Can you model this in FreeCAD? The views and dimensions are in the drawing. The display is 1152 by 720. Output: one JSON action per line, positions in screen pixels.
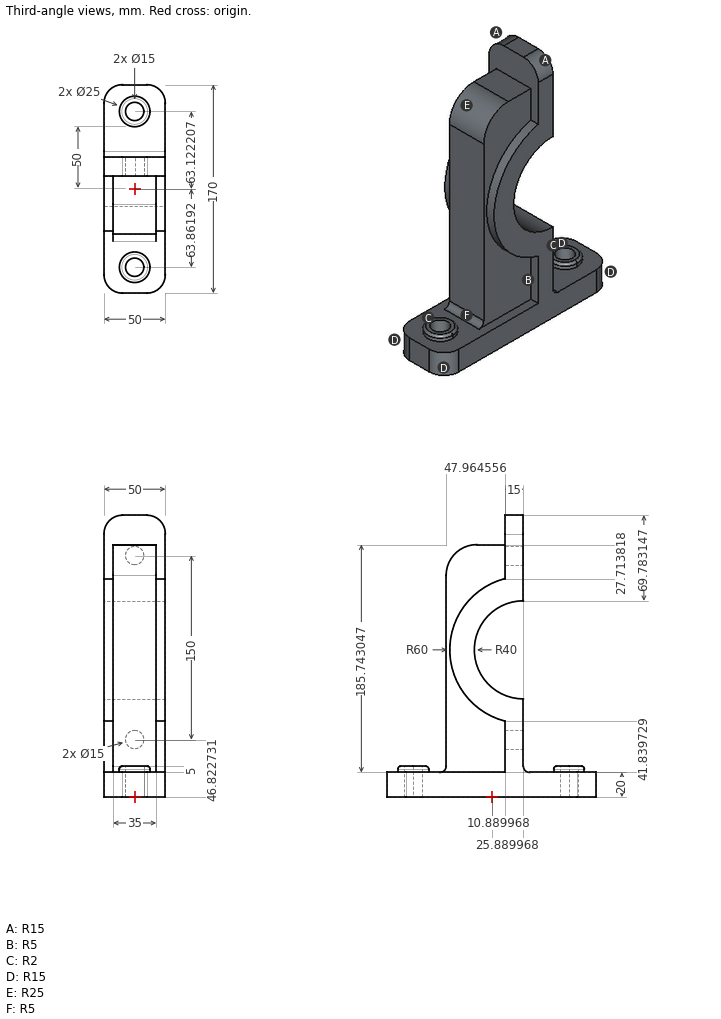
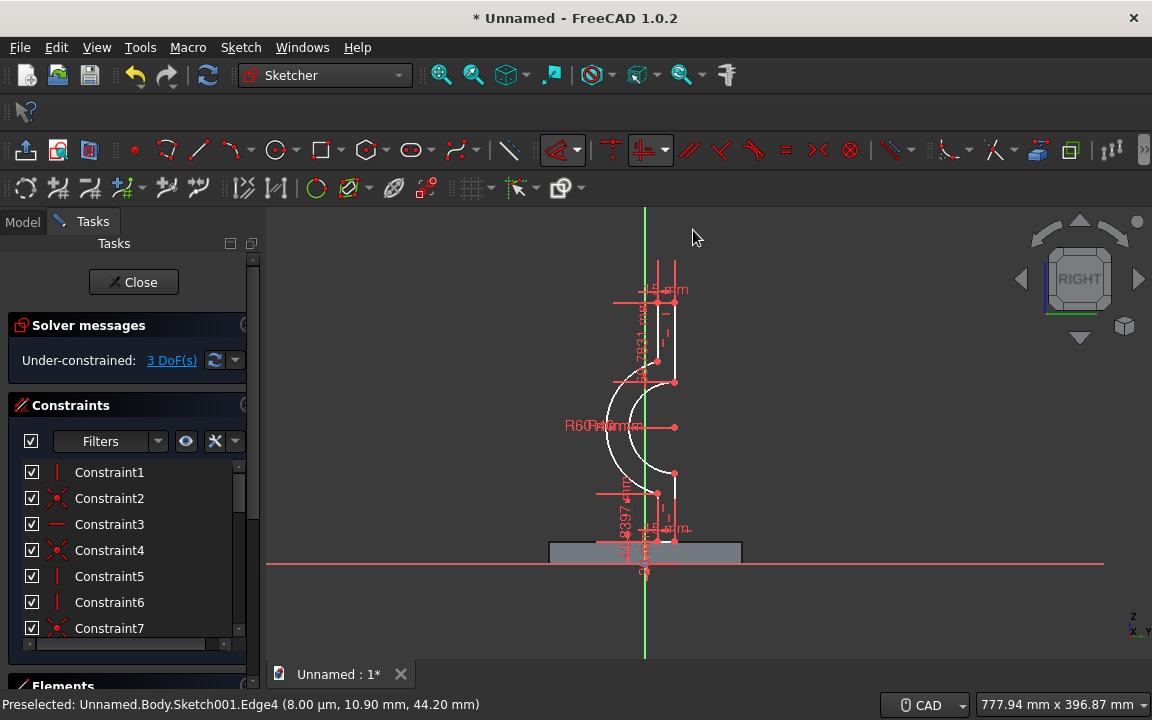
{"action": "scroll", "coordinate": [675, 382], "scroll_direction": "up", "scroll_amount": 2}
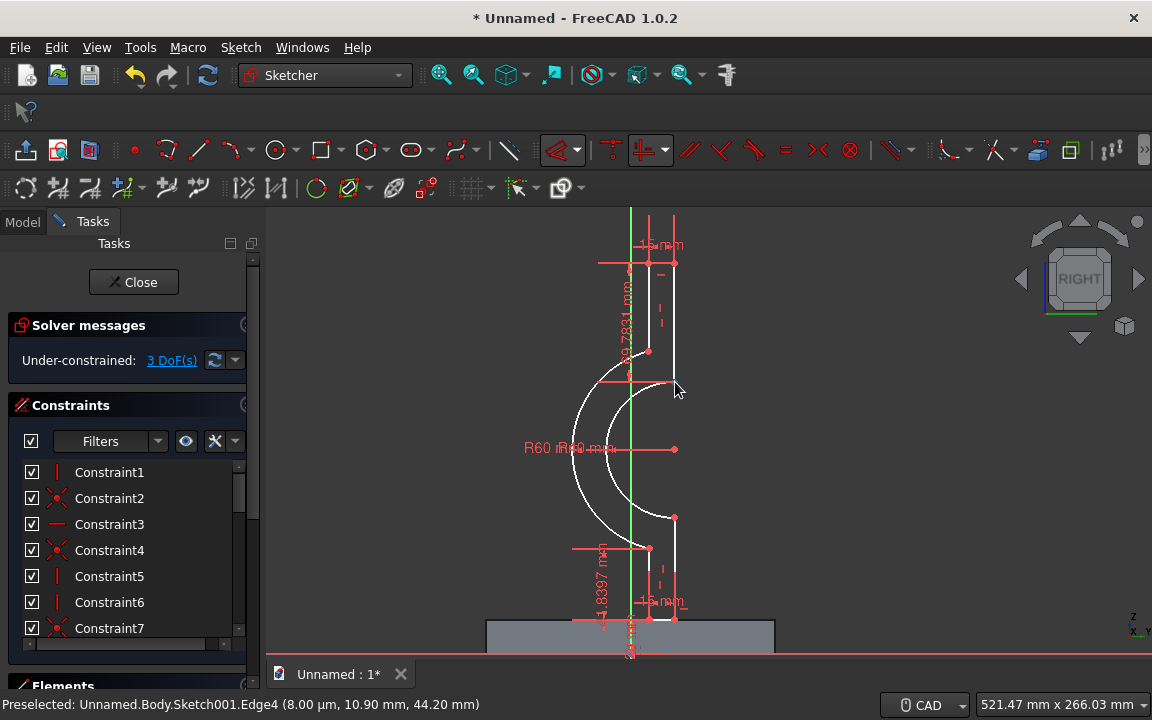
{"action": "left_click", "coordinate": [674, 382]}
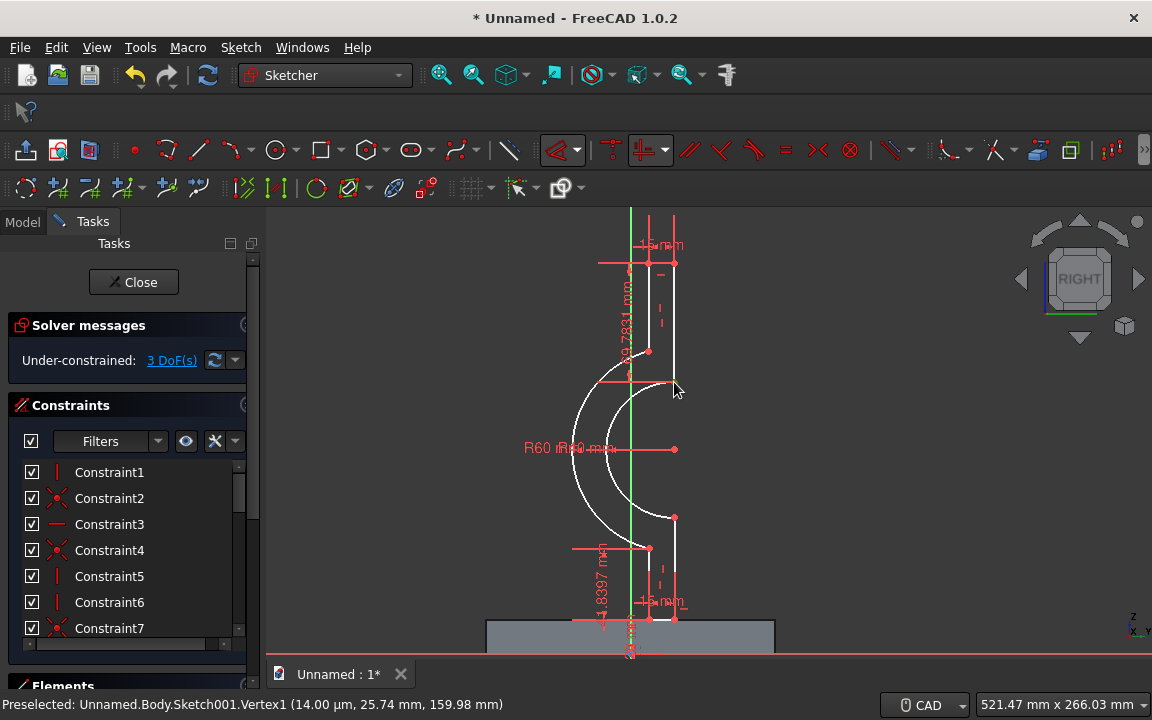
{"action": "key", "text": "l"}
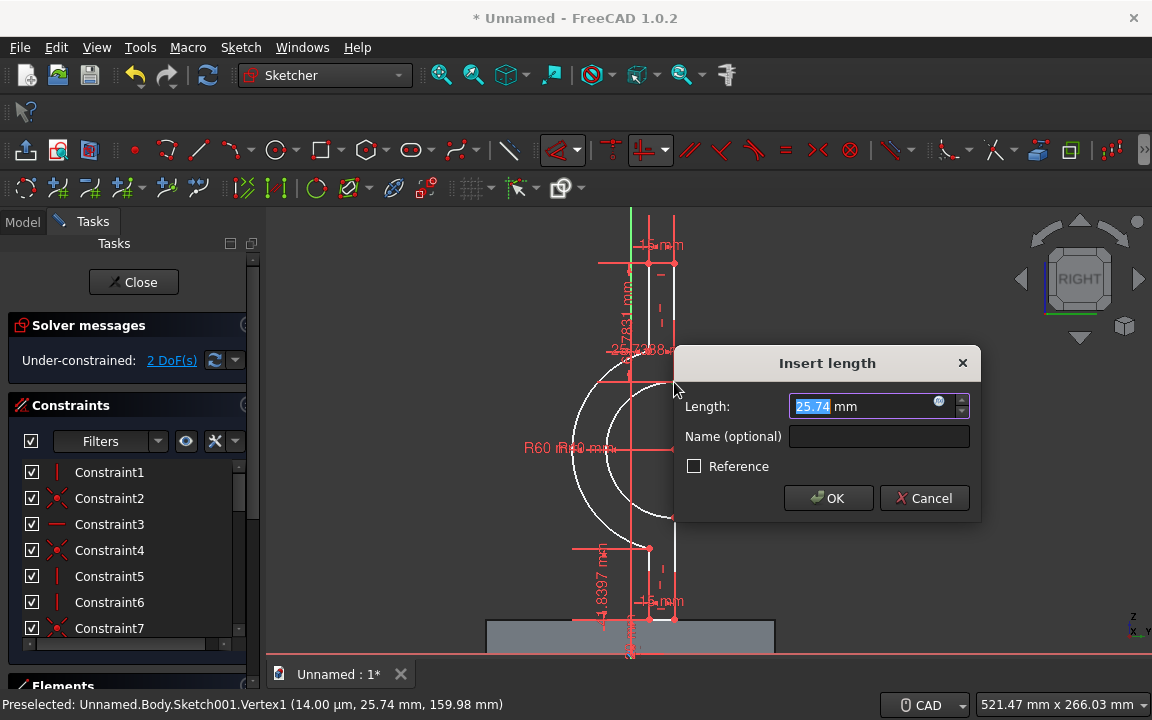
{"action": "type", "text": "25.889968"}
{"action": "key", "text": "Return"}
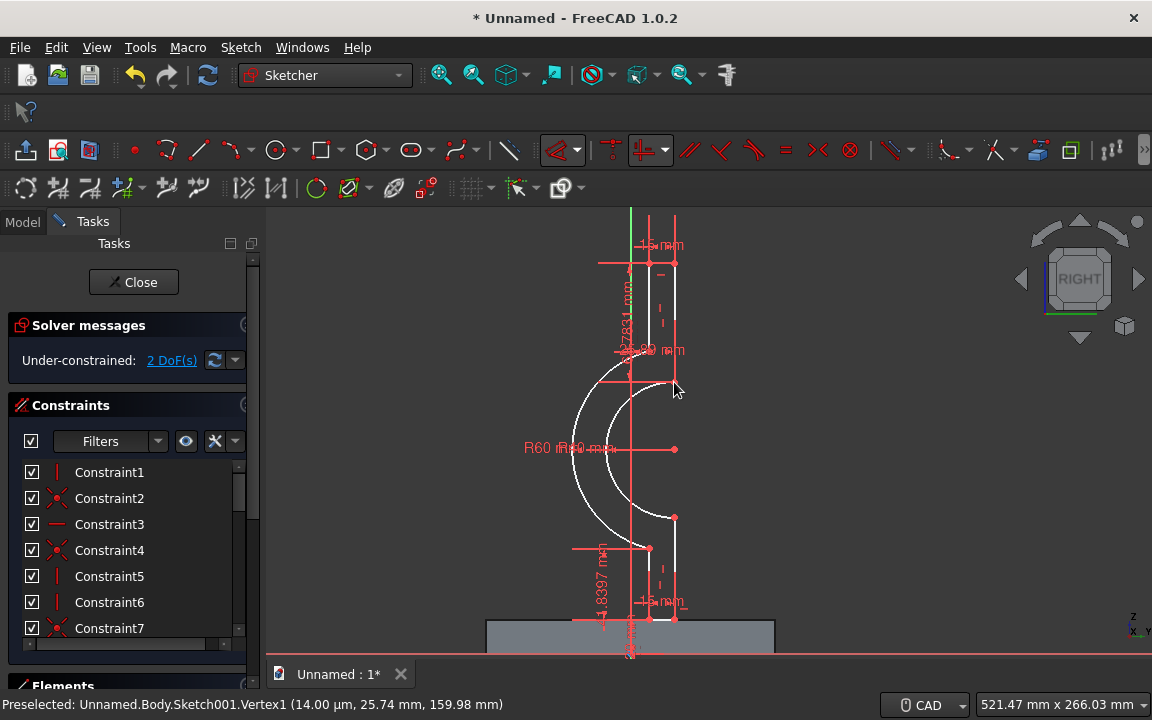
{"action": "scroll", "coordinate": [649, 549], "scroll_direction": "up", "scroll_amount": 4}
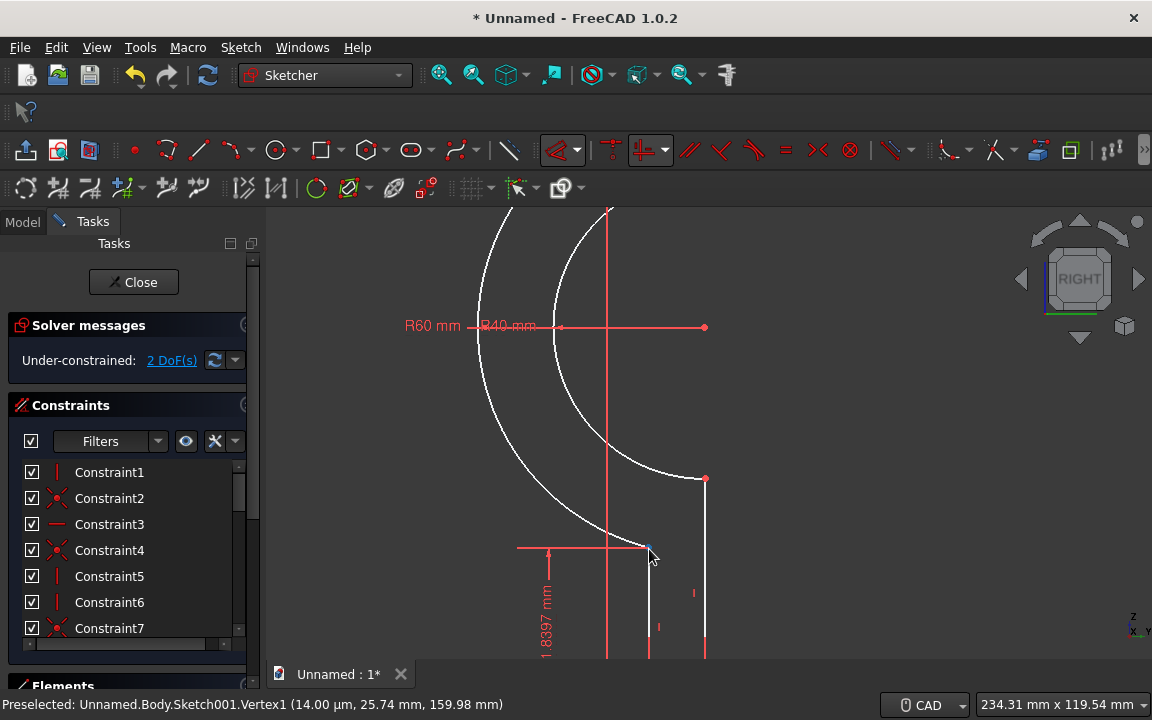
{"action": "left_click", "coordinate": [649, 548]}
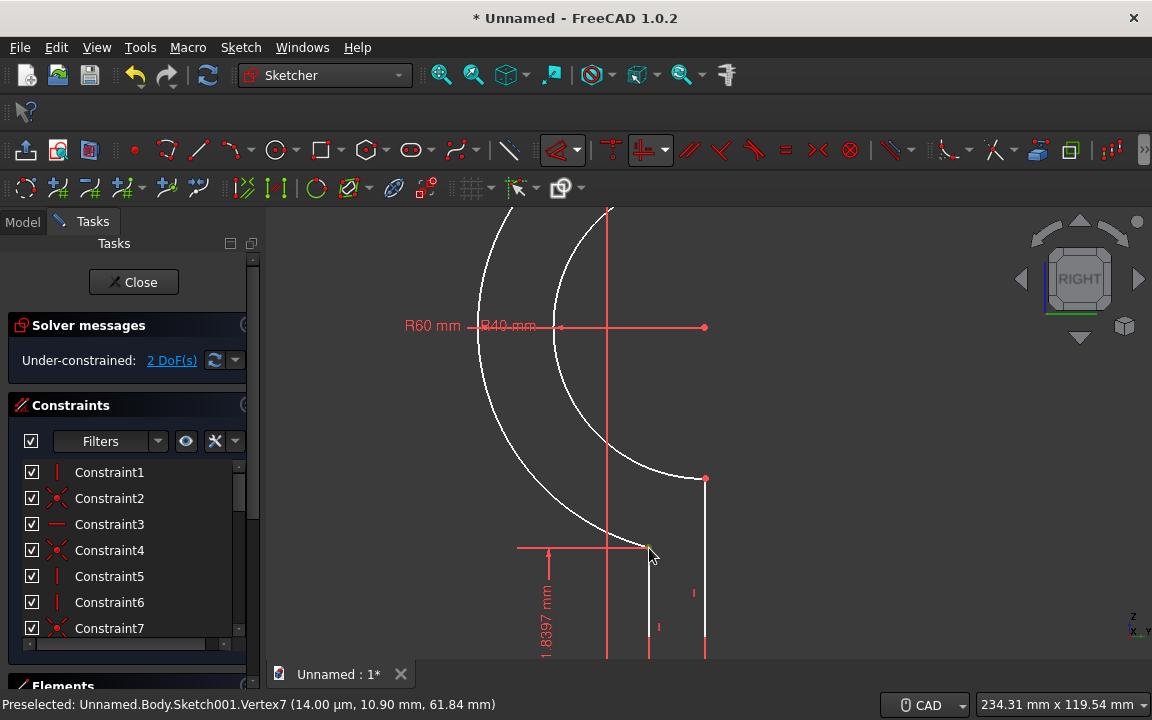
{"action": "key", "text": "l"}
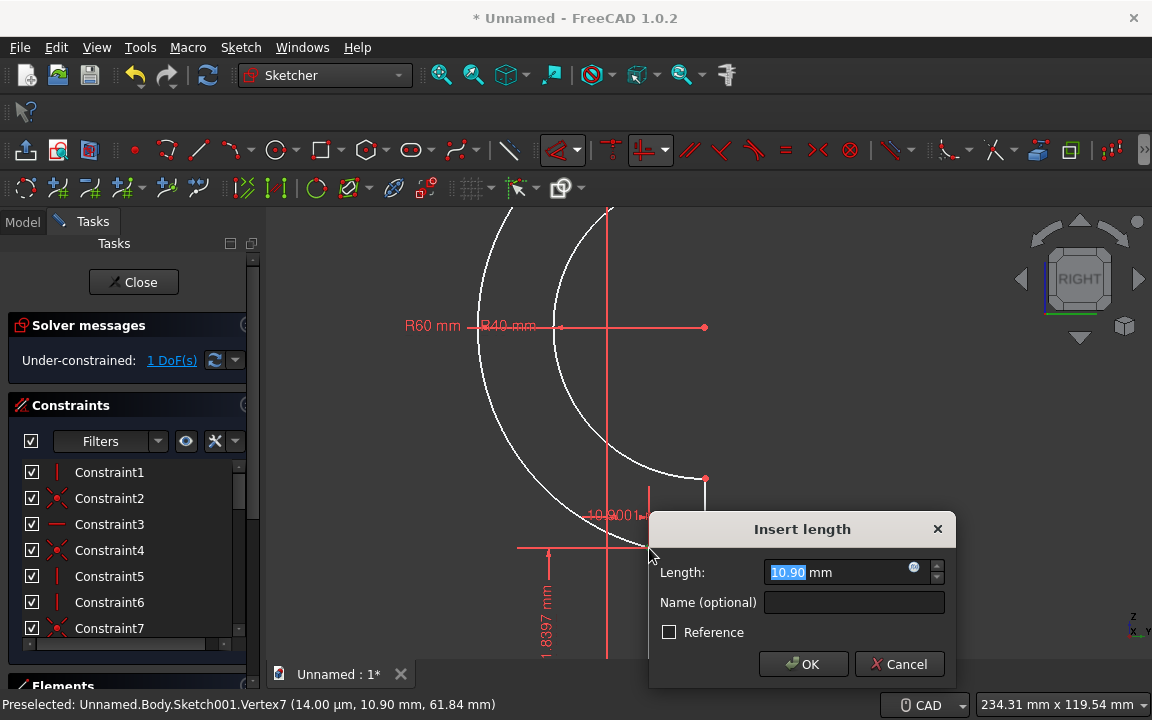
{"action": "type", "text": "10.889968"}
{"action": "key", "text": "Return"}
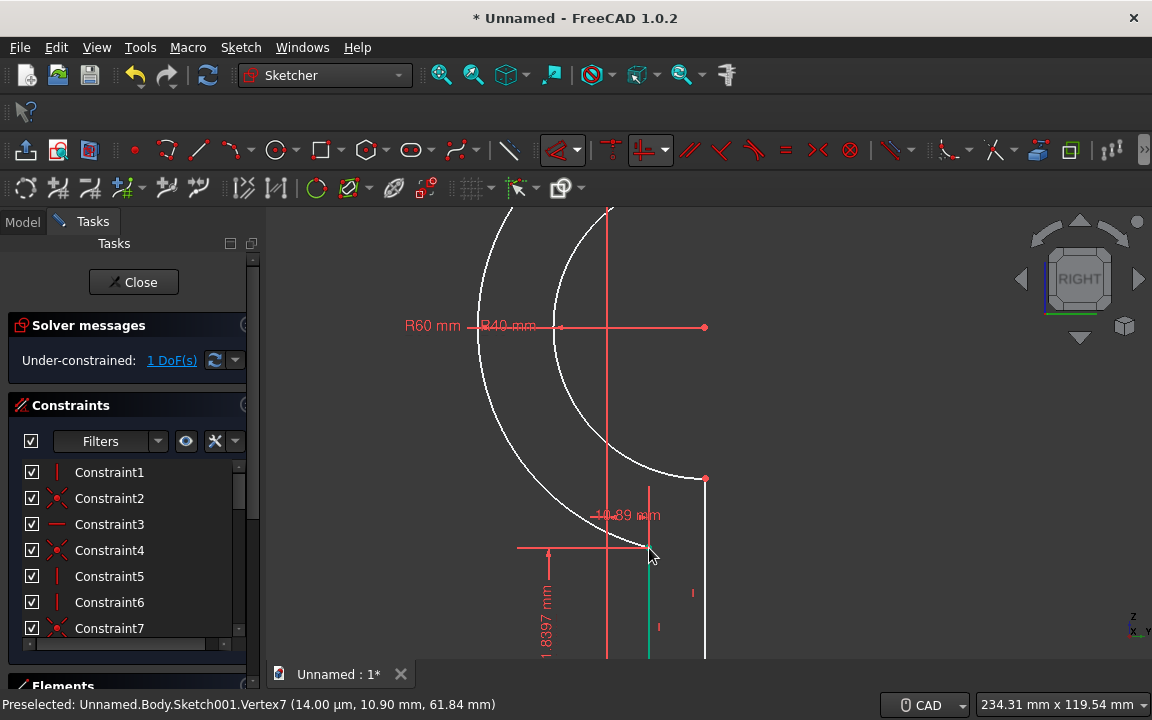
{"action": "left_click", "coordinate": [705, 328]}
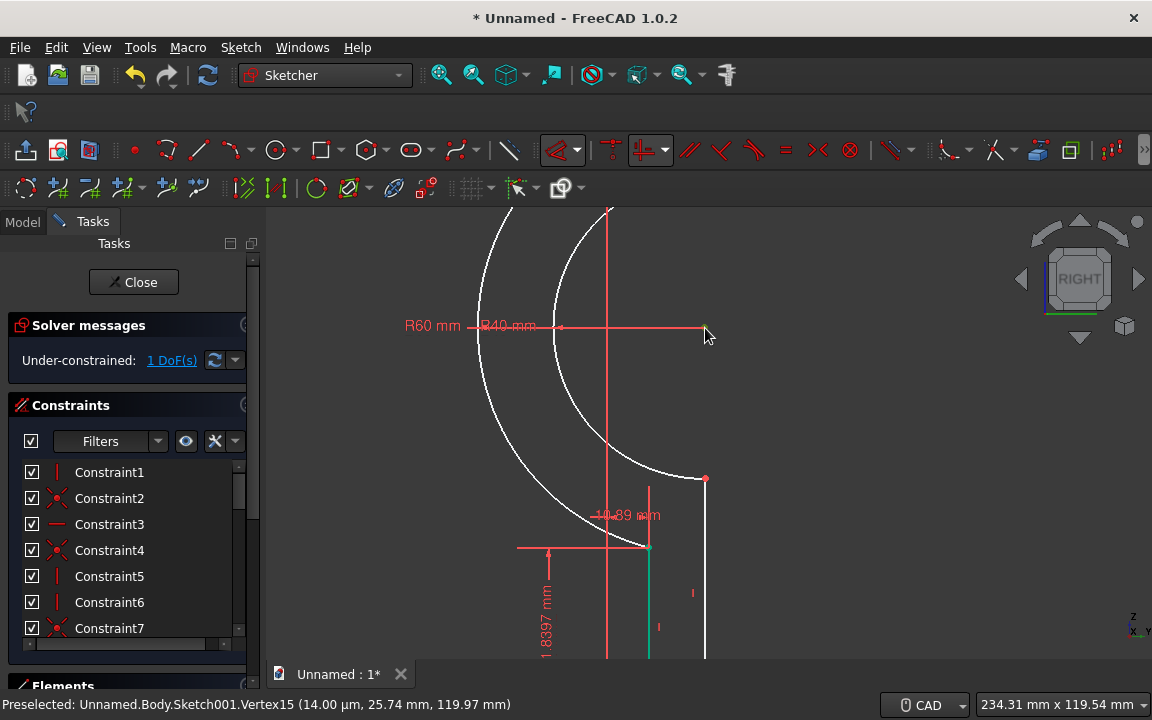
{"action": "key", "text": "l"}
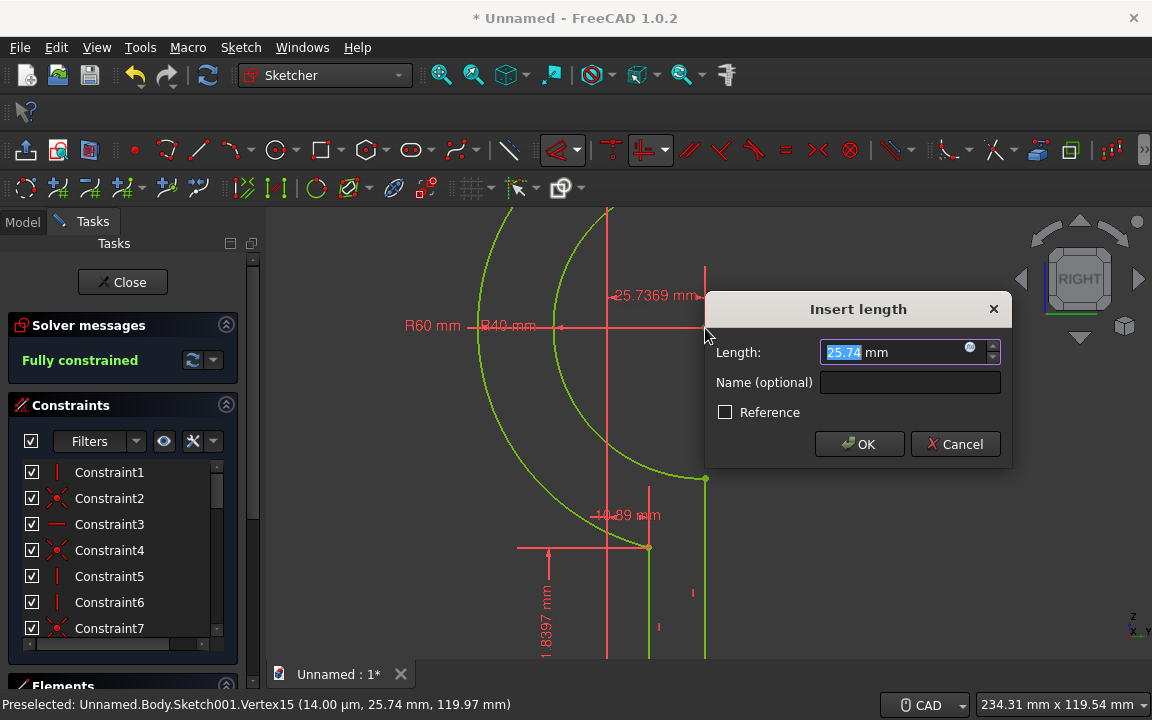
{"action": "type", "text": "25.889968"}
{"action": "key", "text": "Return"}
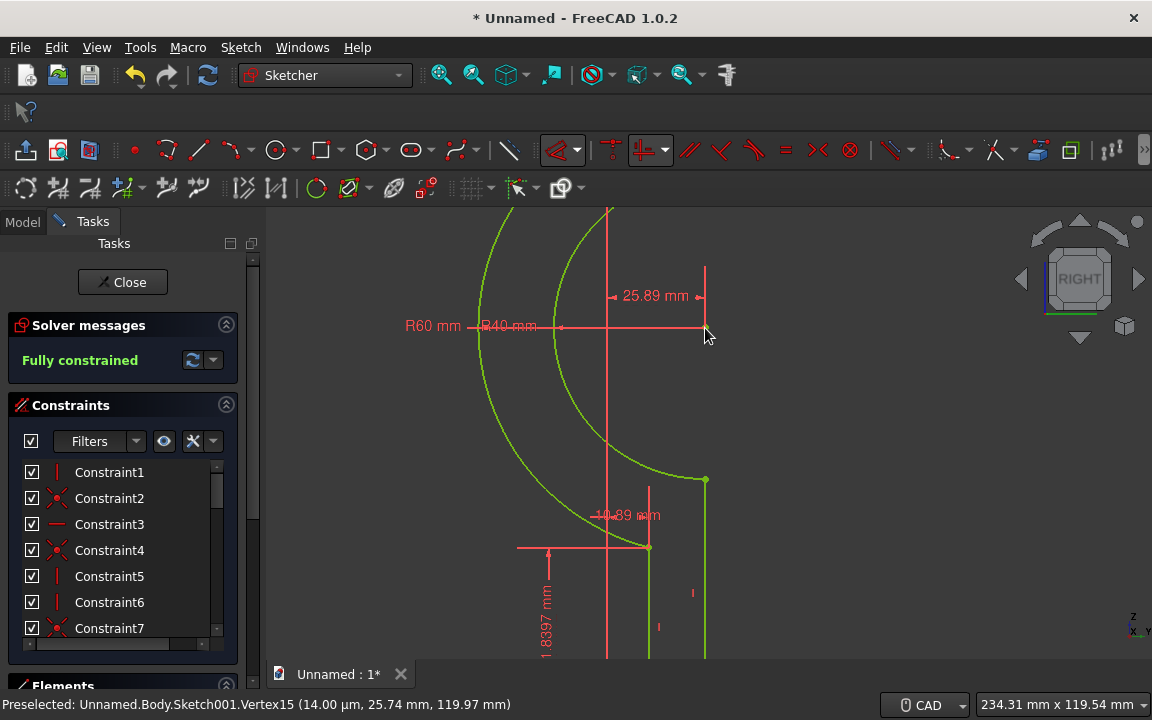
{"action": "left_click", "coordinate": [123, 282]}